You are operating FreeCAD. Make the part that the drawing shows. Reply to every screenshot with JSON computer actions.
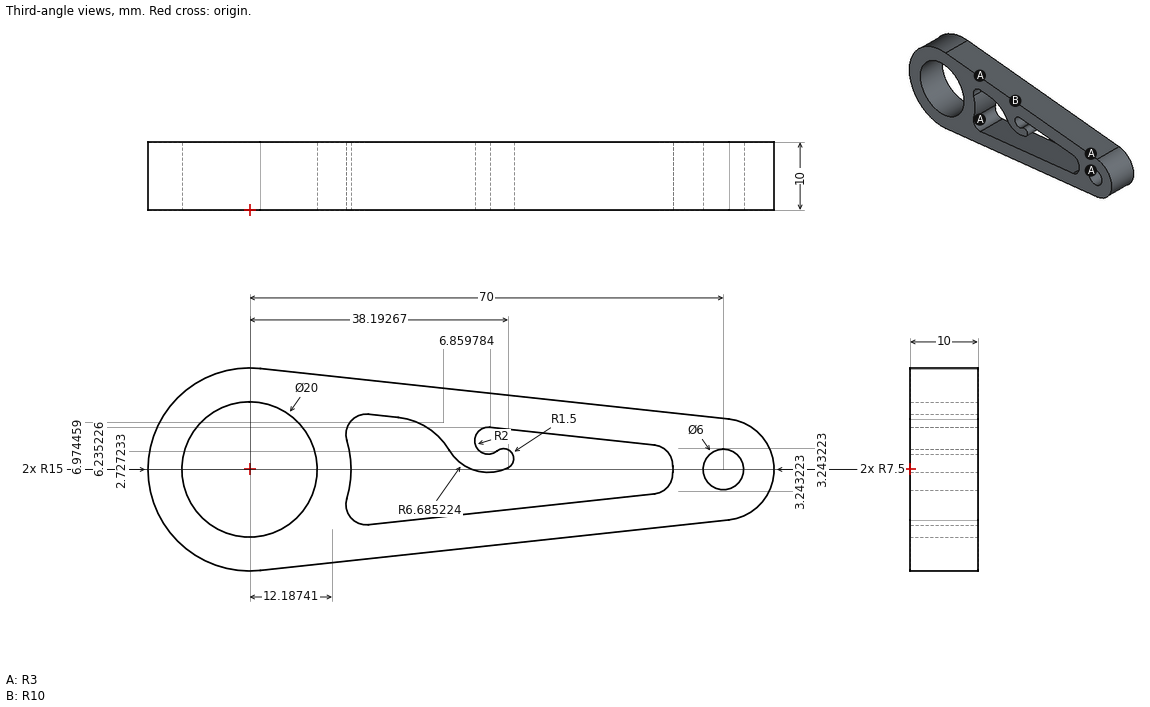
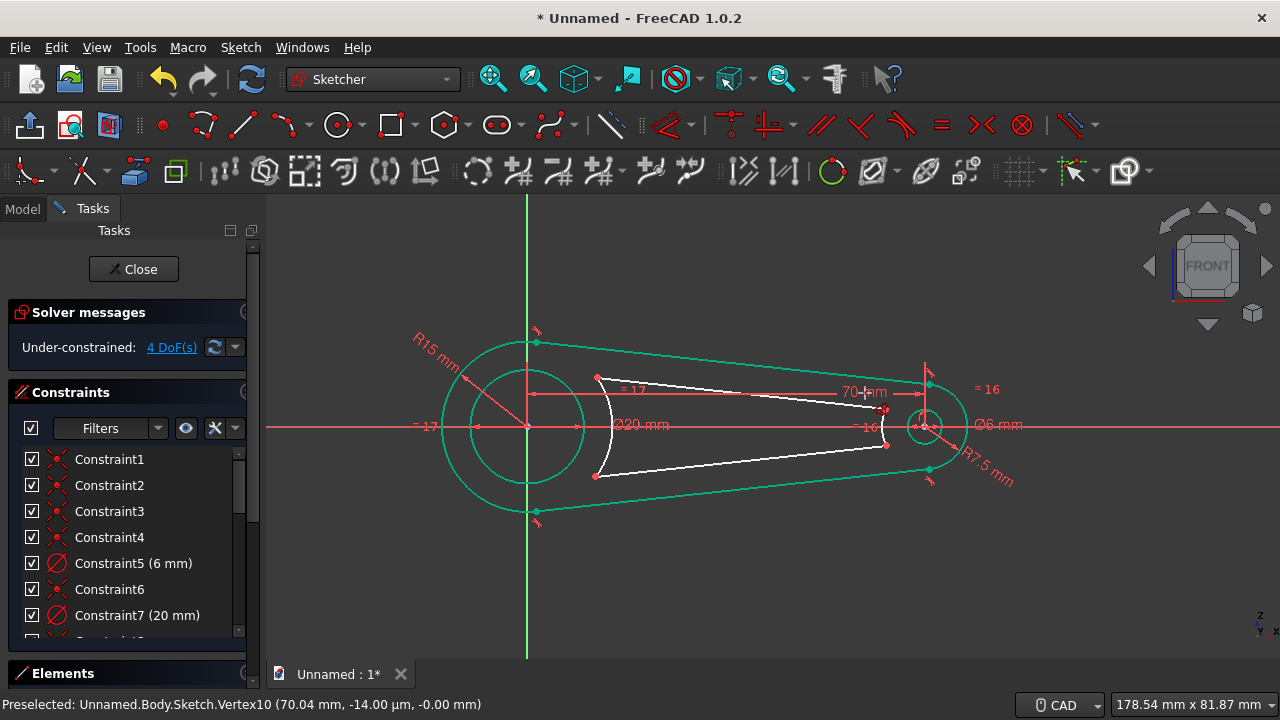
{"action": "left_click", "coordinate": [596, 477]}
{"action": "left_click", "coordinate": [546, 393]}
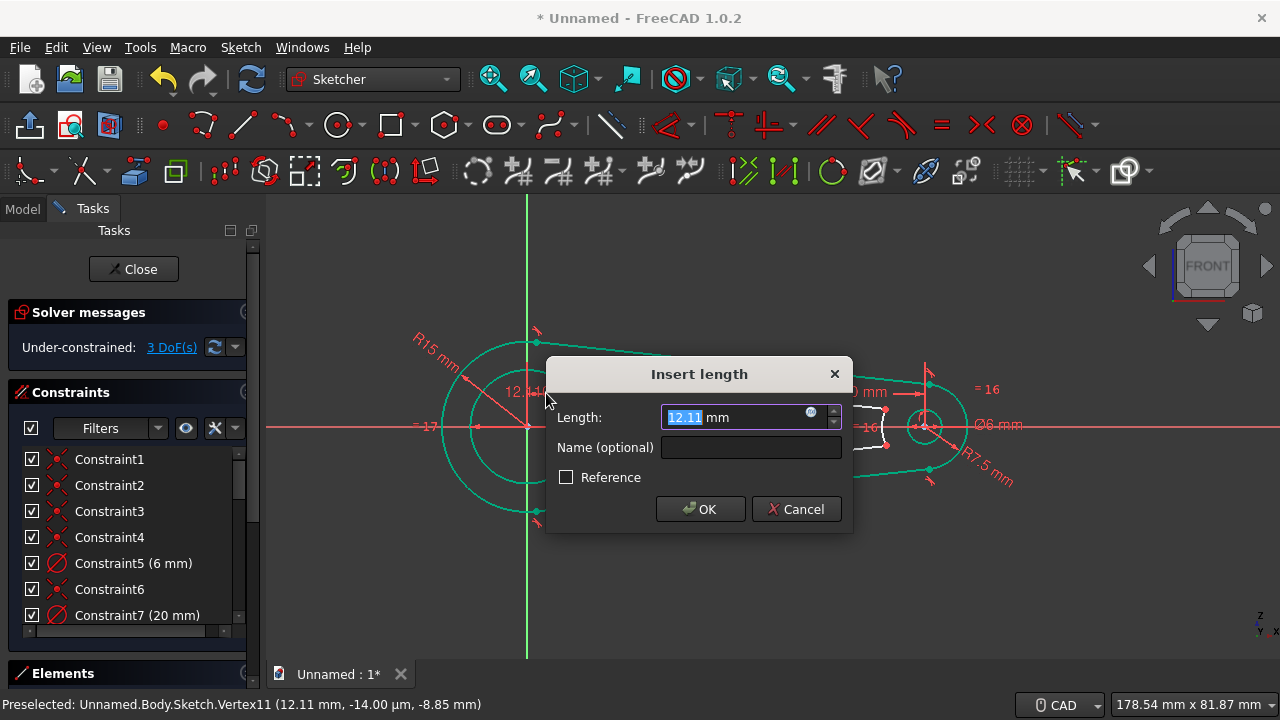
{"action": "type", "text": "12.18741"}
{"action": "key", "text": "Return"}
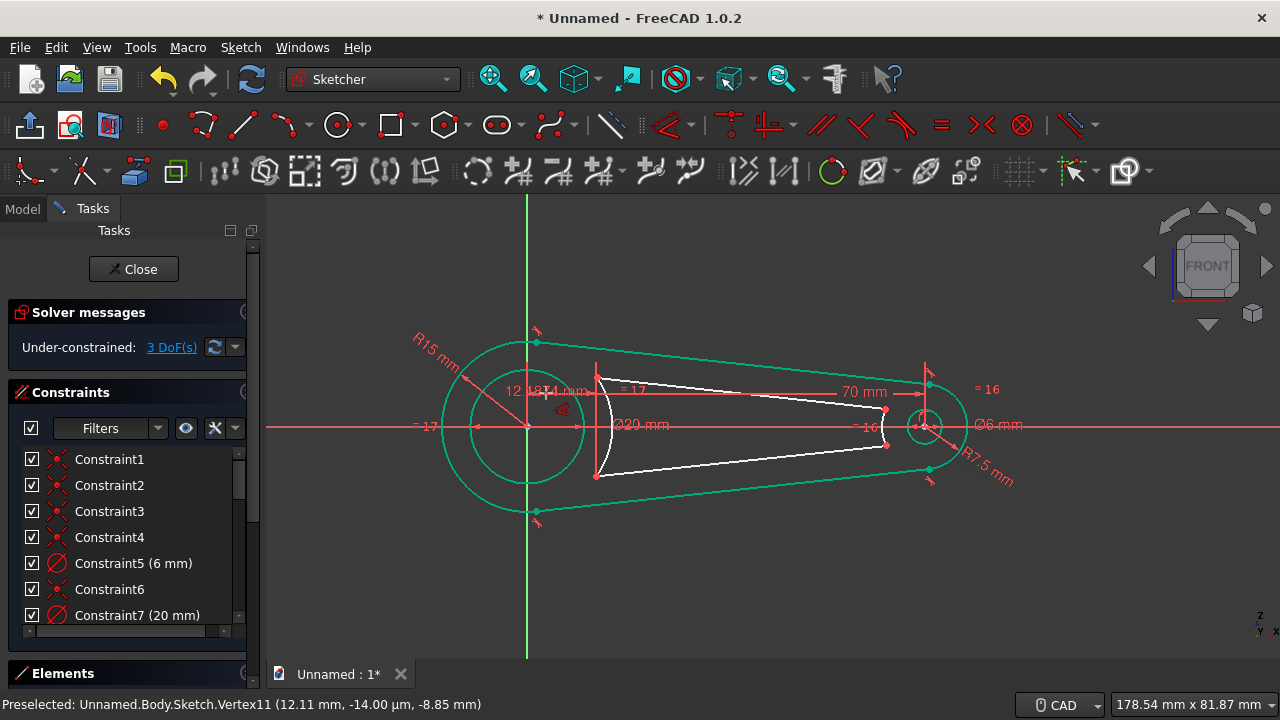
{"action": "scroll", "coordinate": [887, 446], "scroll_direction": "up", "scroll_amount": 4}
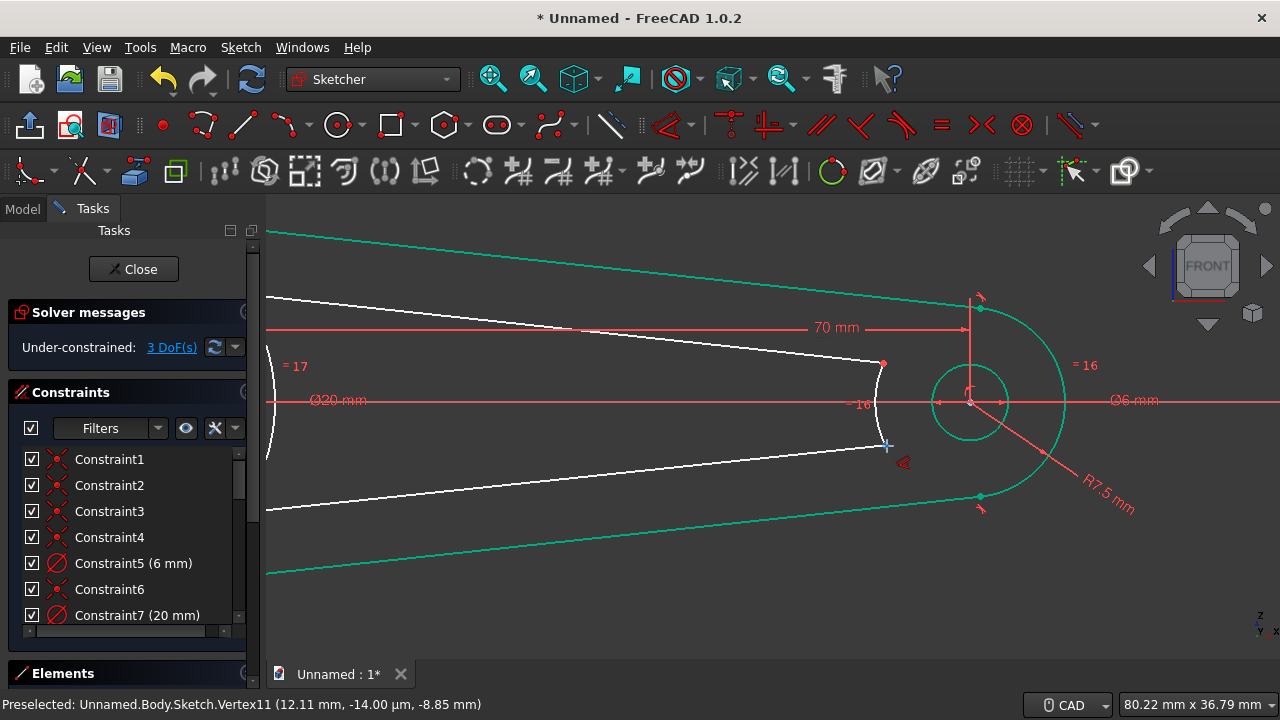
{"action": "left_click", "coordinate": [886, 445]}
{"action": "left_click", "coordinate": [920, 424]}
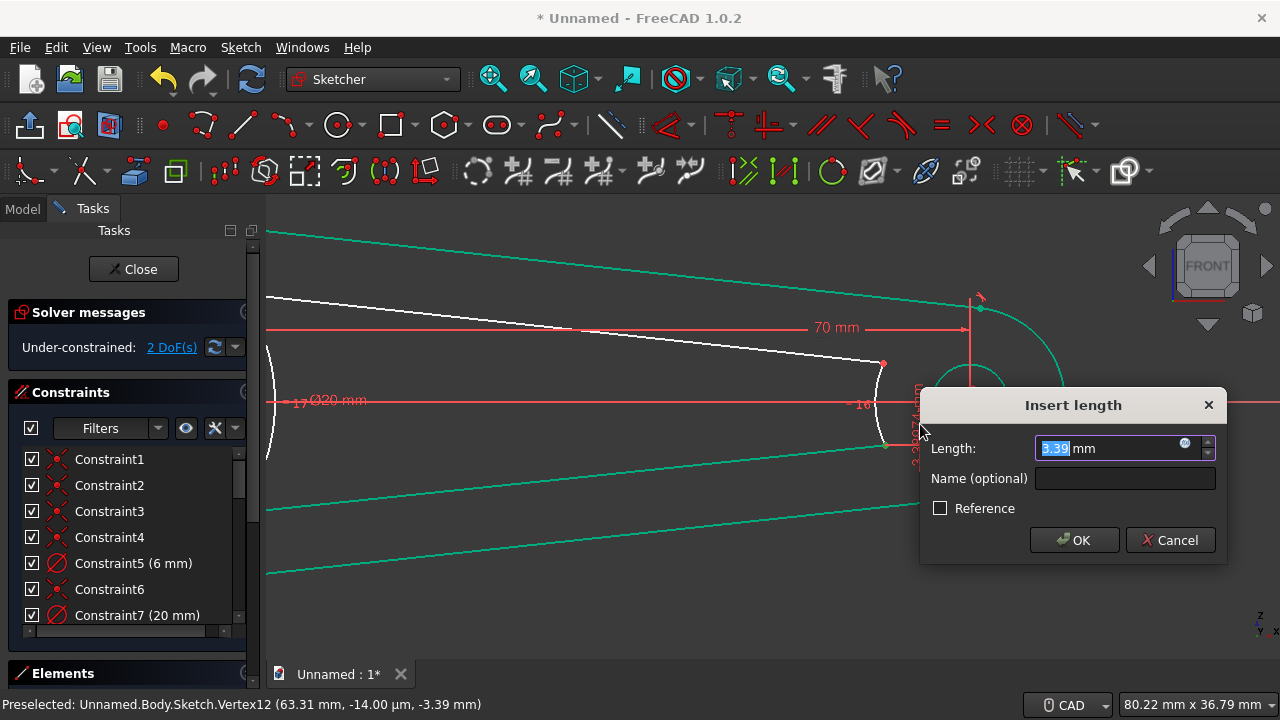
{"action": "type", "text": "3.243223"}
{"action": "key", "text": "Return"}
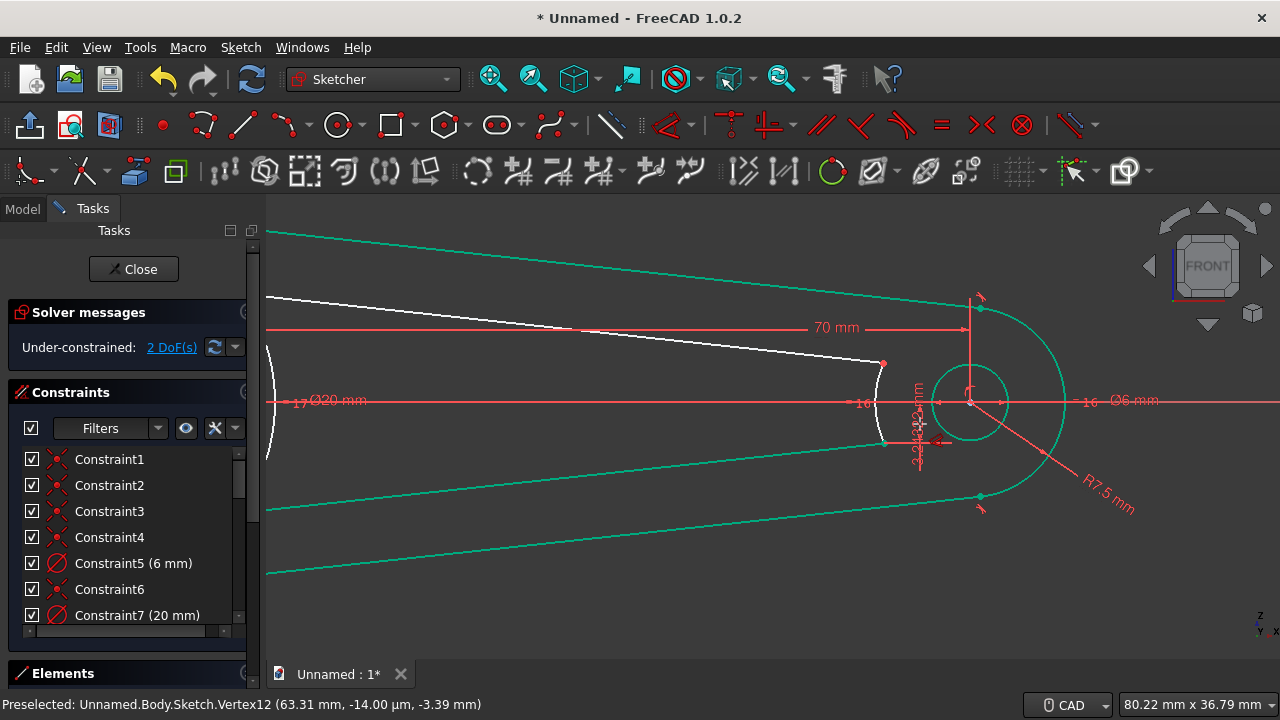
{"action": "left_click", "coordinate": [884, 363]}
{"action": "left_click", "coordinate": [918, 383]}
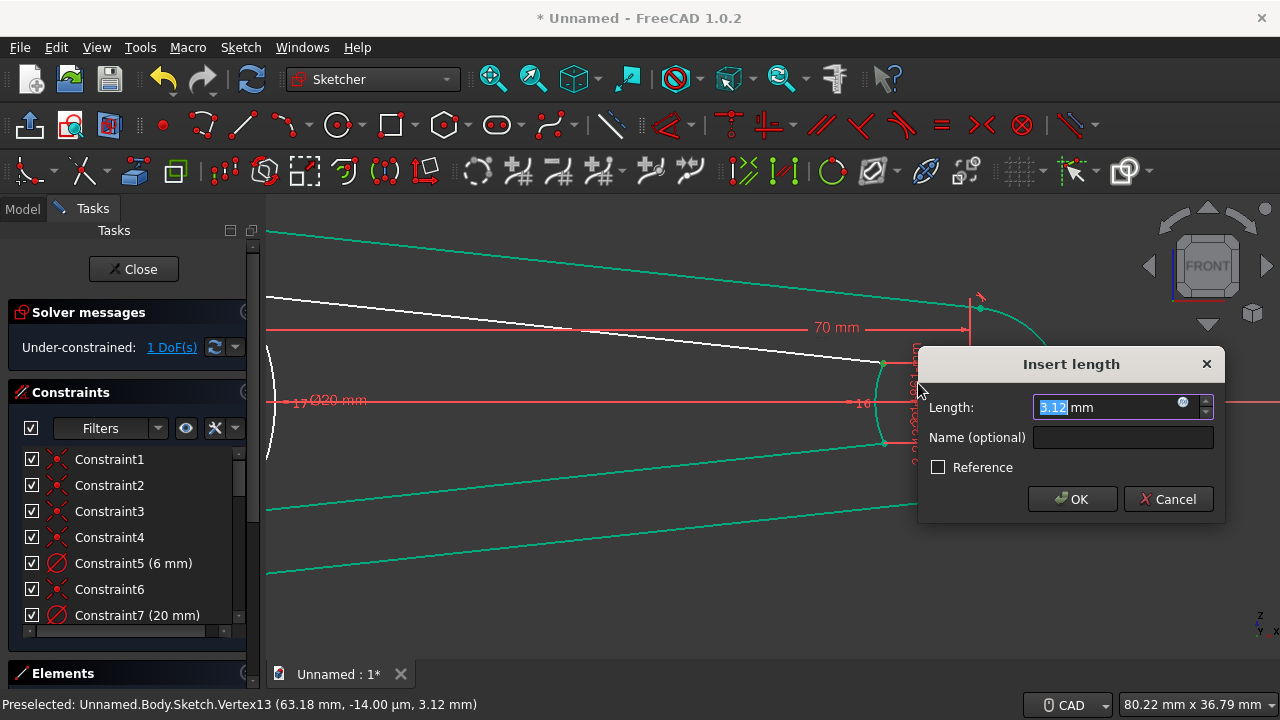
{"action": "type", "text": "3.243223"}
{"action": "key", "text": "Return"}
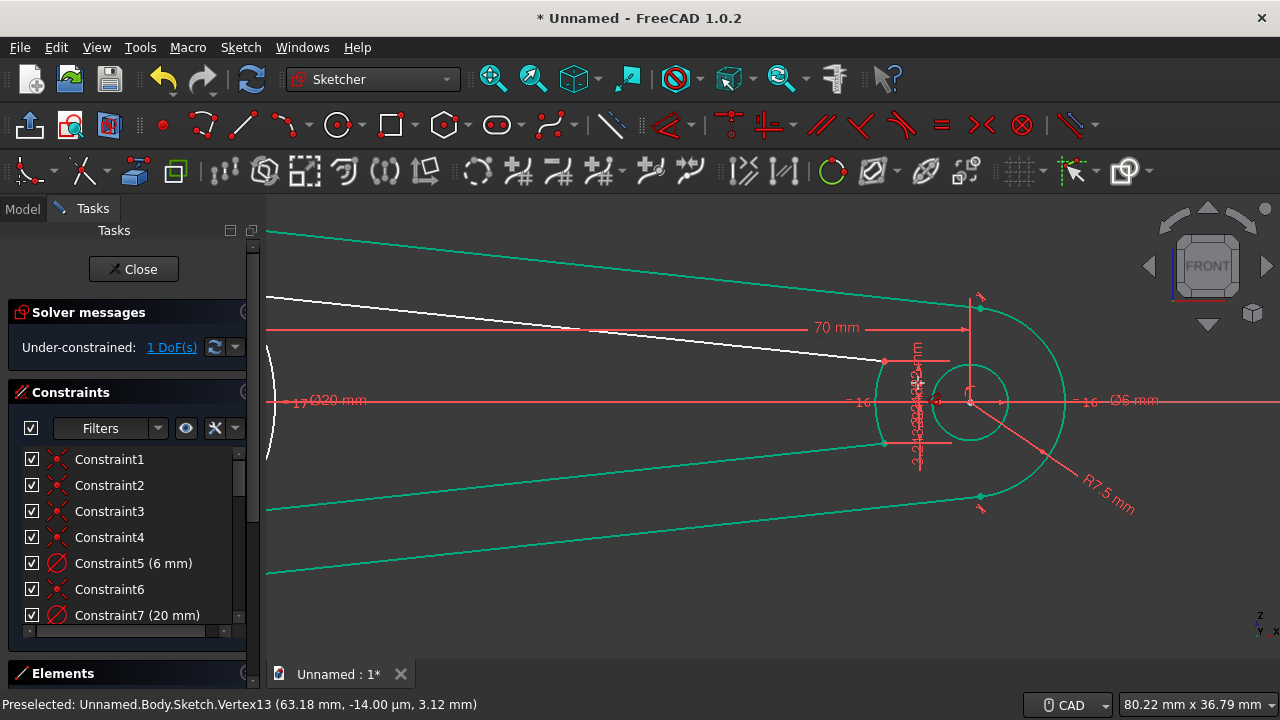
{"action": "scroll", "coordinate": [887, 446], "scroll_direction": "down", "scroll_amount": 4}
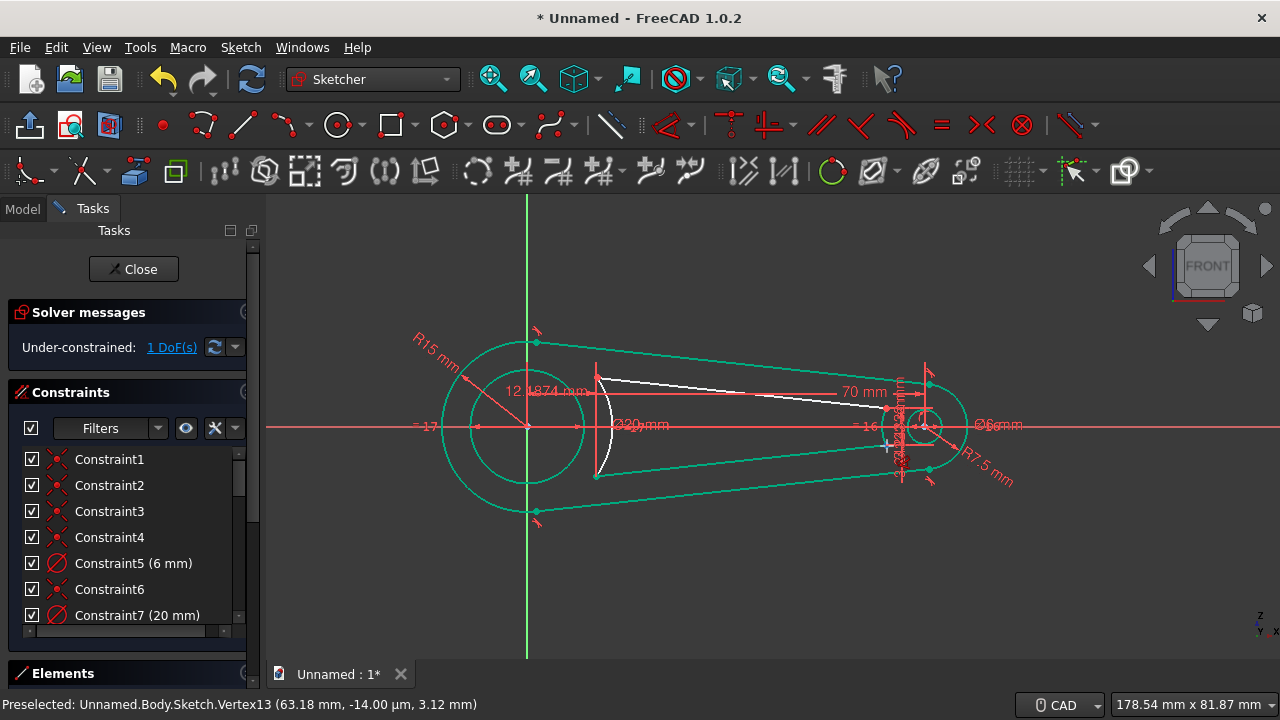
{"action": "left_click", "coordinate": [597, 378]}
{"action": "left_click", "coordinate": [546, 461]}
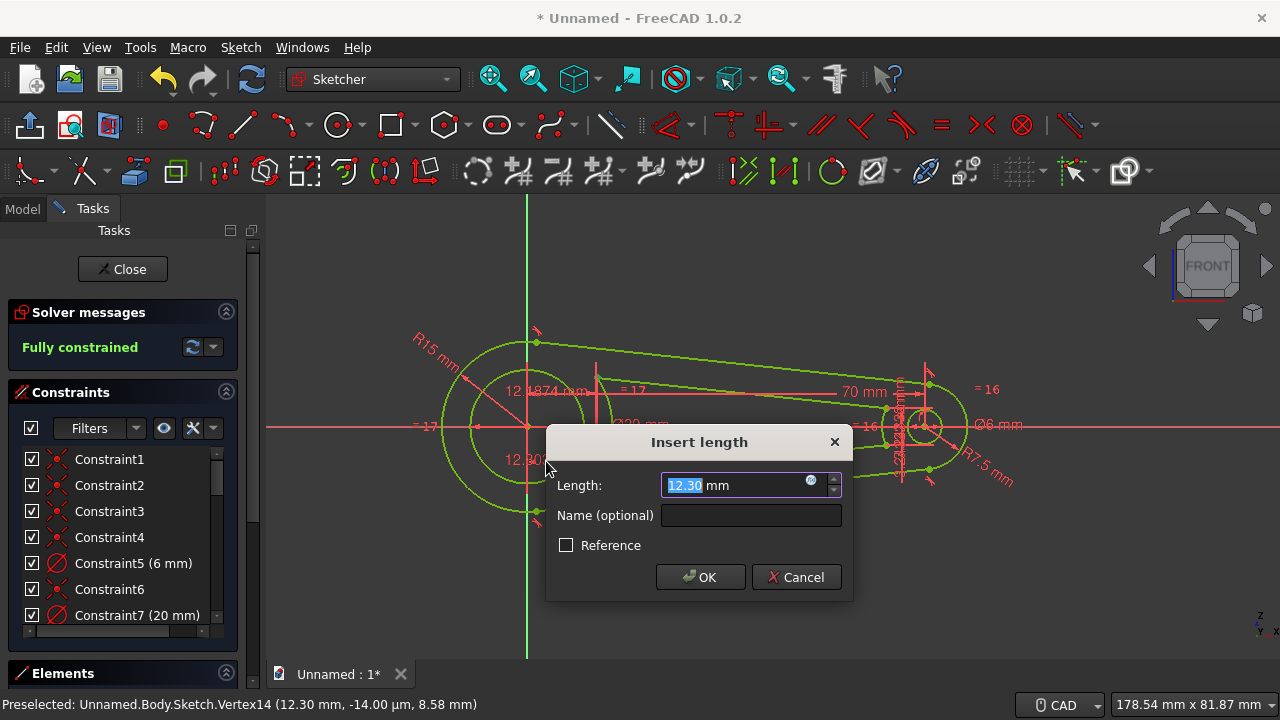
{"action": "type", "text": "12.18741"}
{"action": "key", "text": "Return"}
{"action": "key", "text": "Escape"}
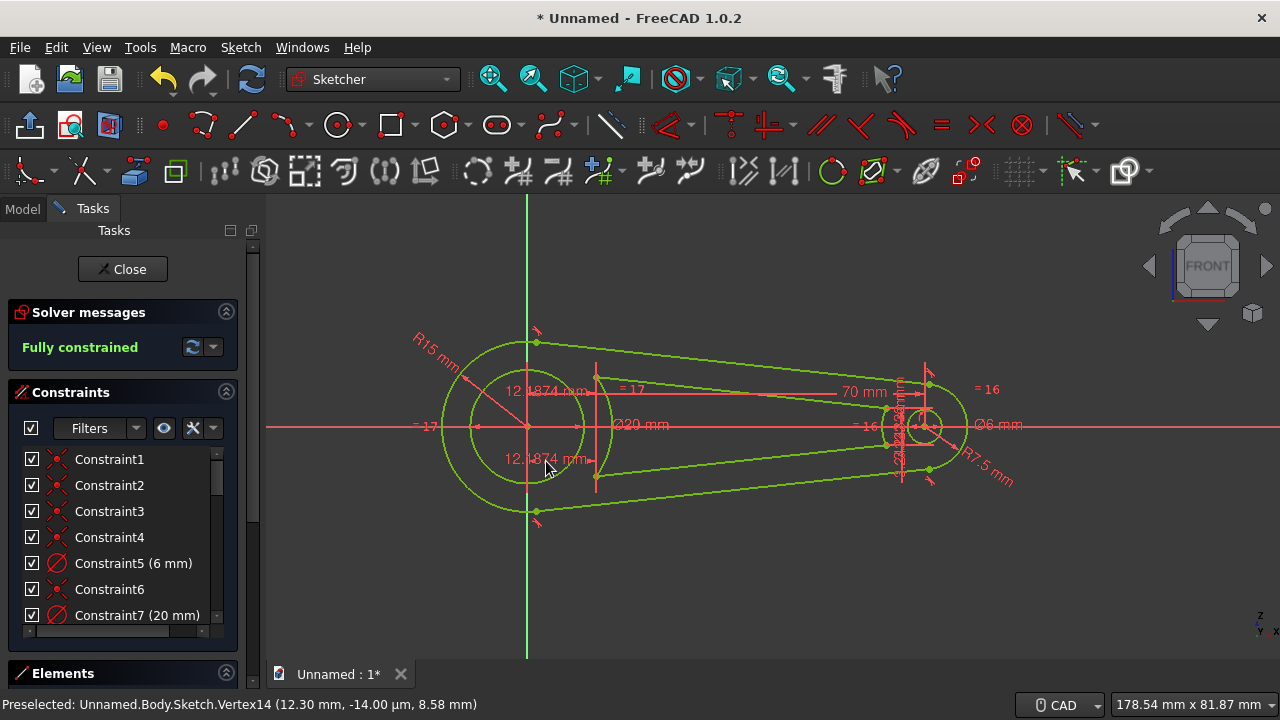
{"action": "left_click", "coordinate": [123, 269]}